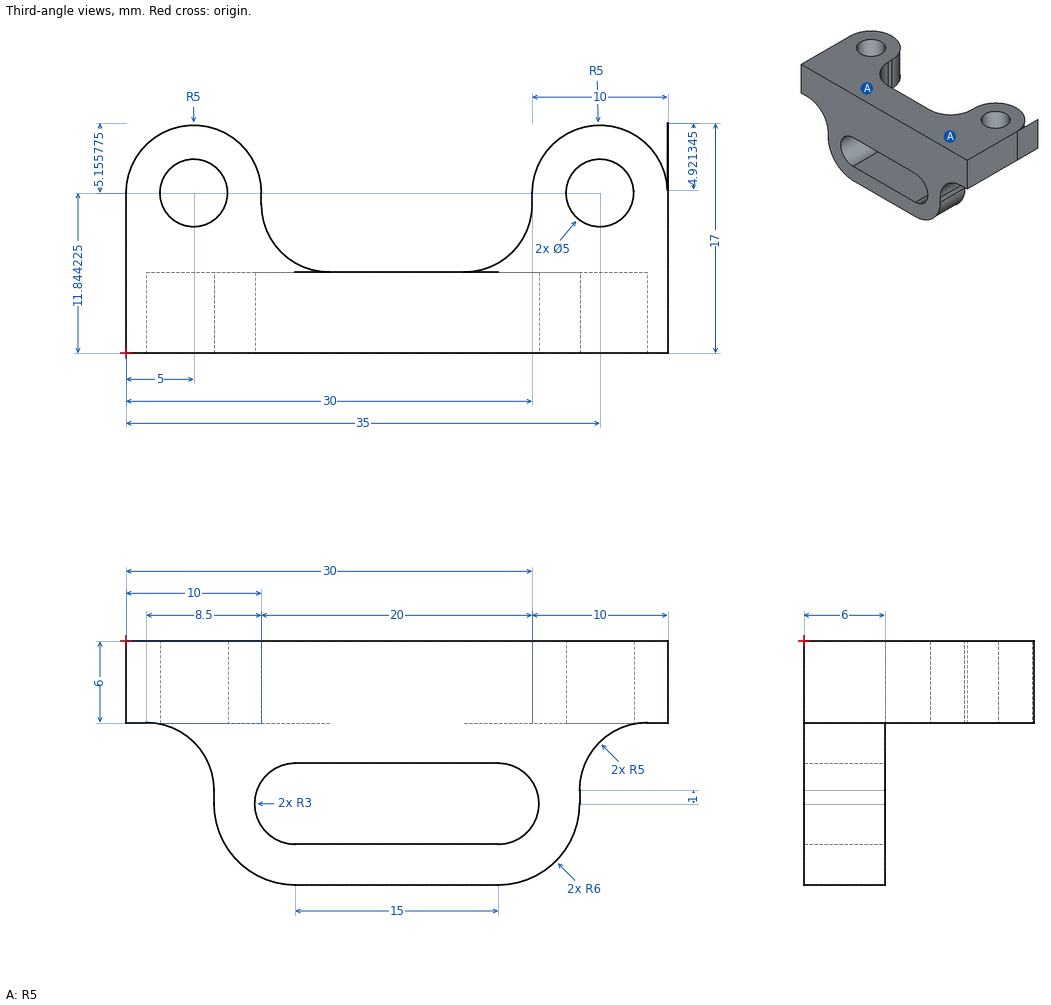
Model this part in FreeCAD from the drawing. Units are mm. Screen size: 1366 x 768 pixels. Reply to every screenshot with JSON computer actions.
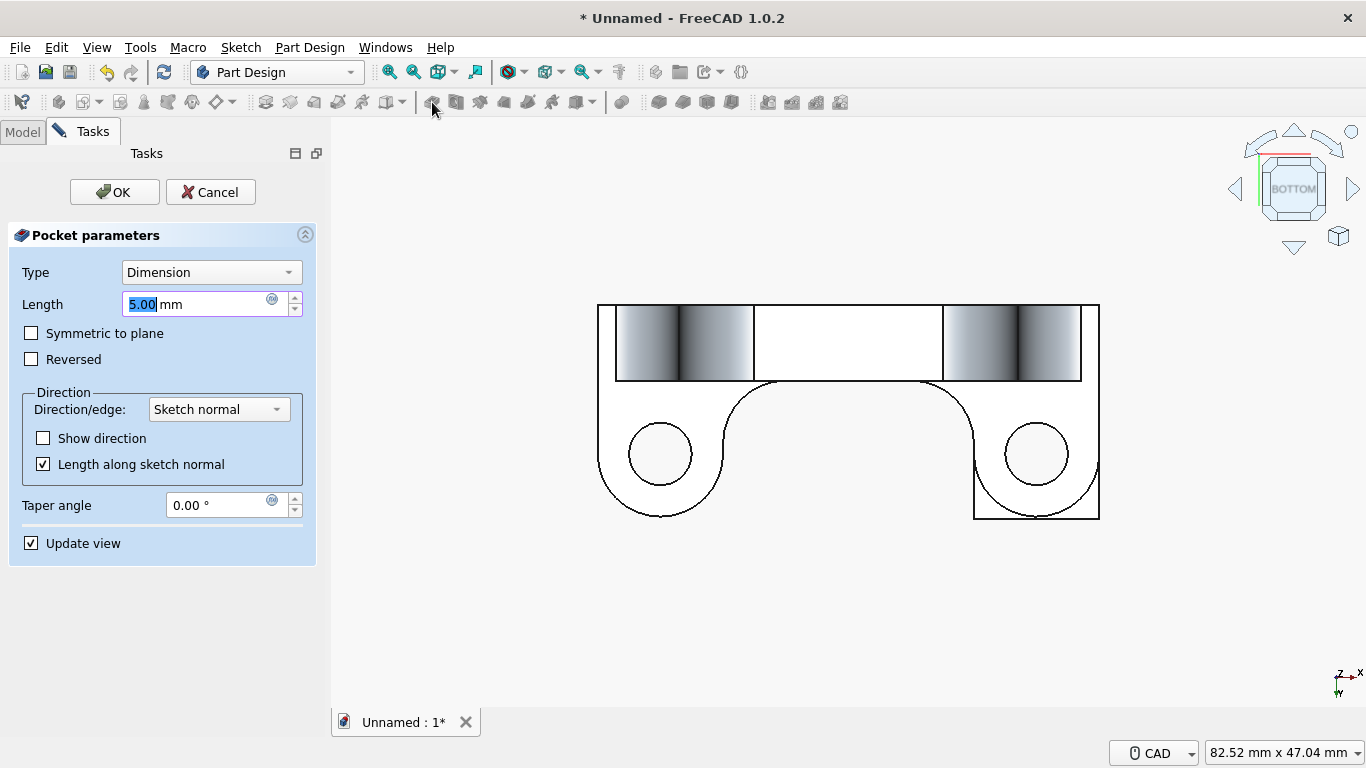
{"action": "type", "text": "17"}
{"action": "key", "text": "Tab"}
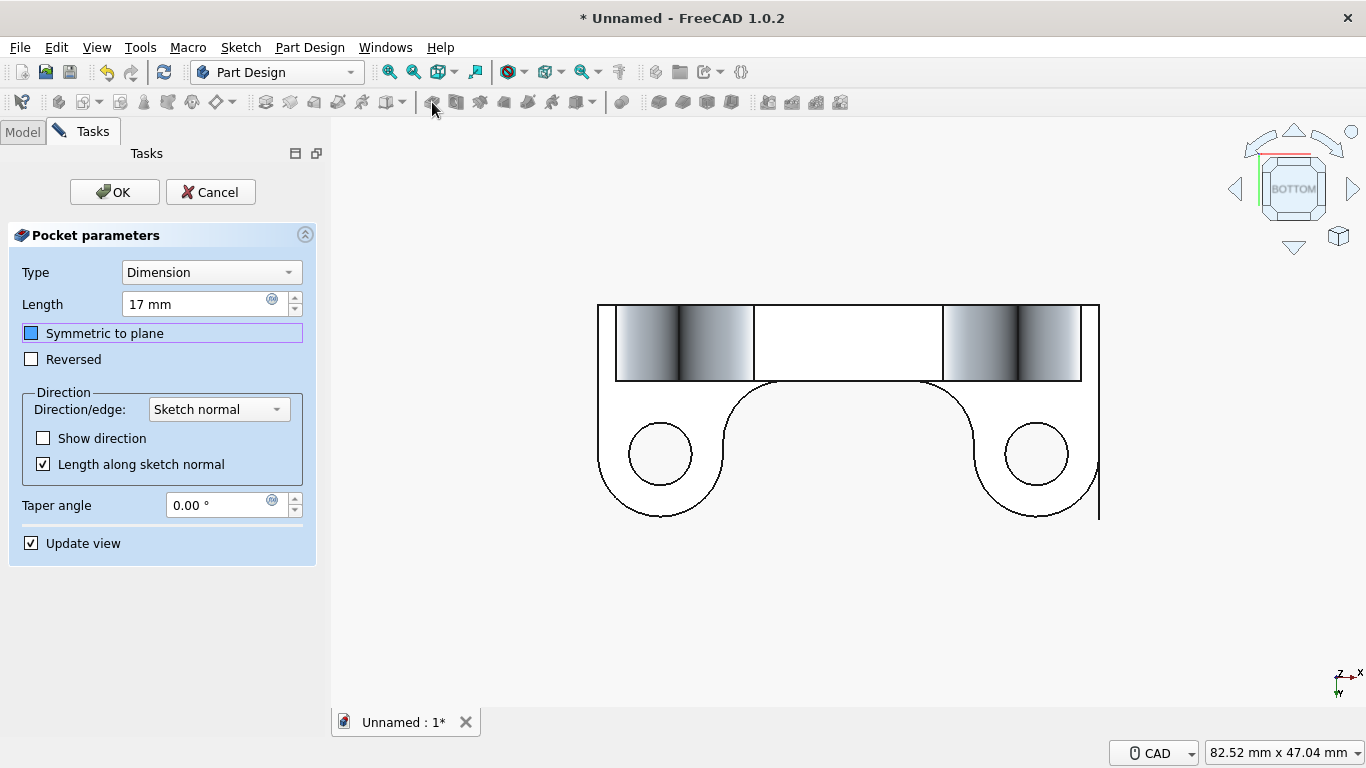
{"action": "left_click", "coordinate": [115, 192]}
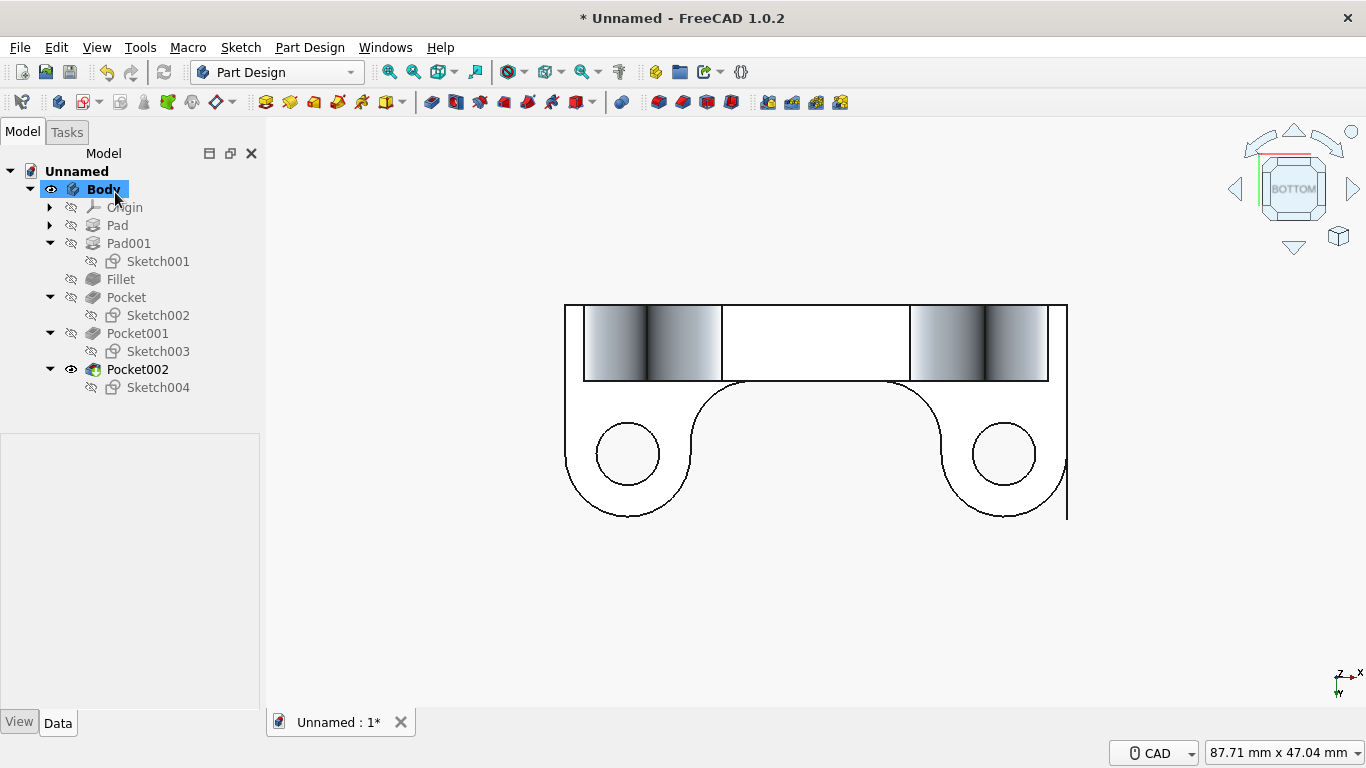
{"action": "key", "text": "0"}